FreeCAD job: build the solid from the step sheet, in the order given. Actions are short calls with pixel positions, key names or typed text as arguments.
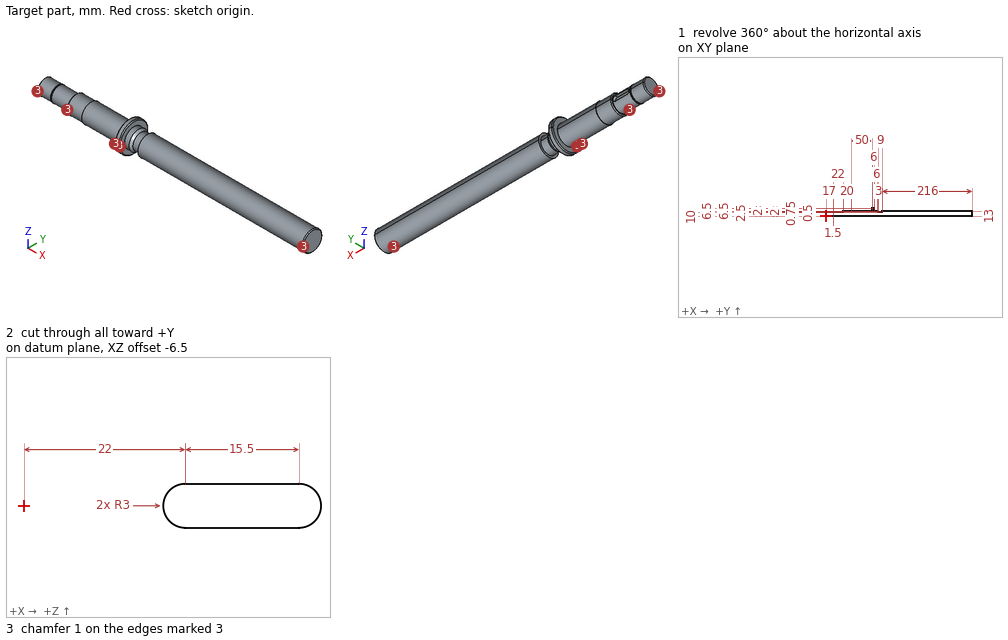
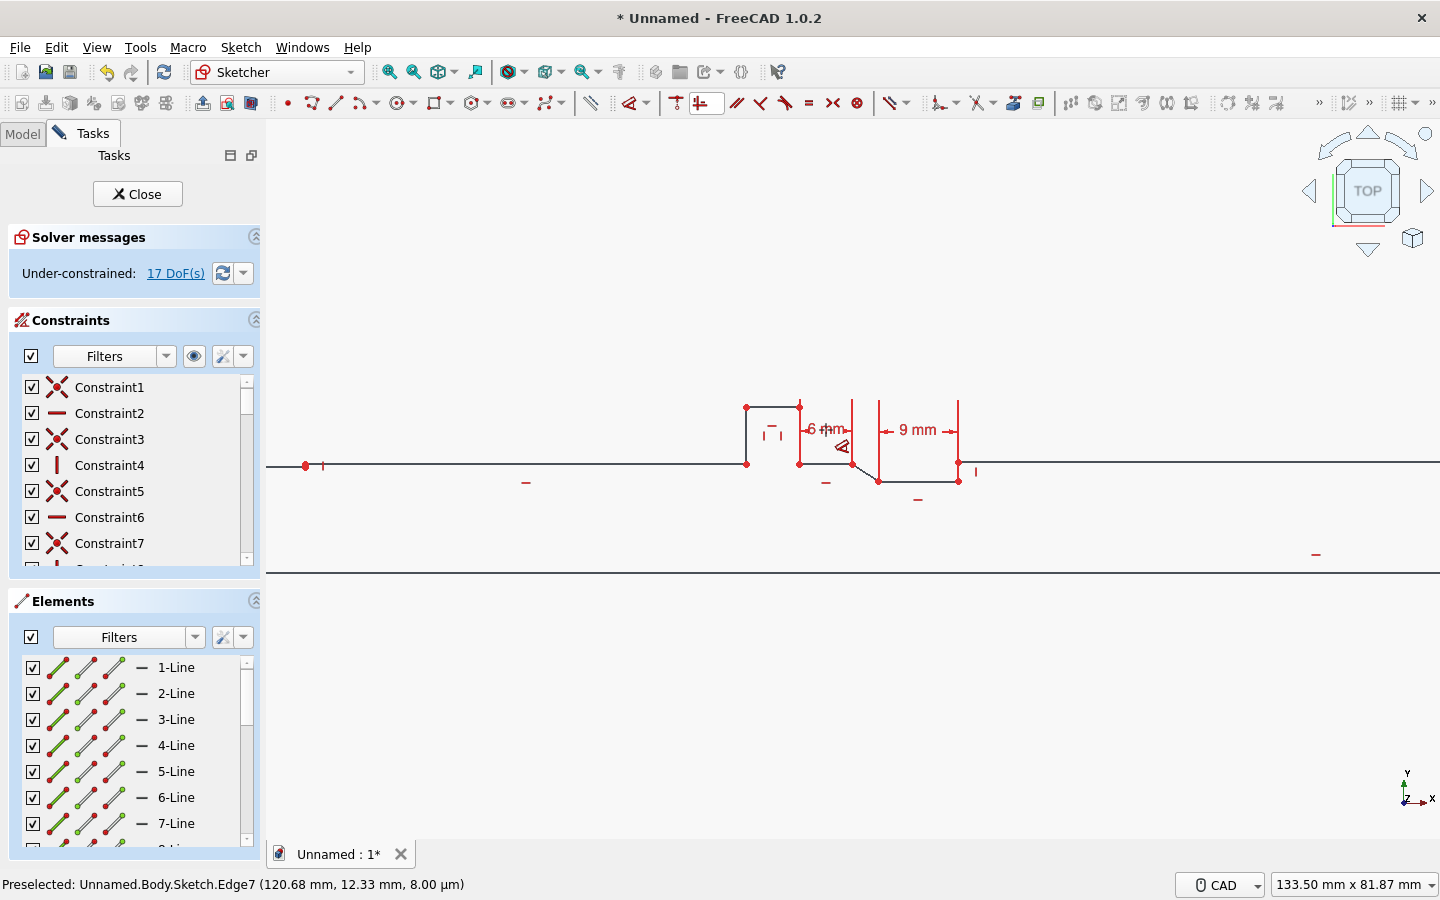
click(784, 407)
click(773, 373)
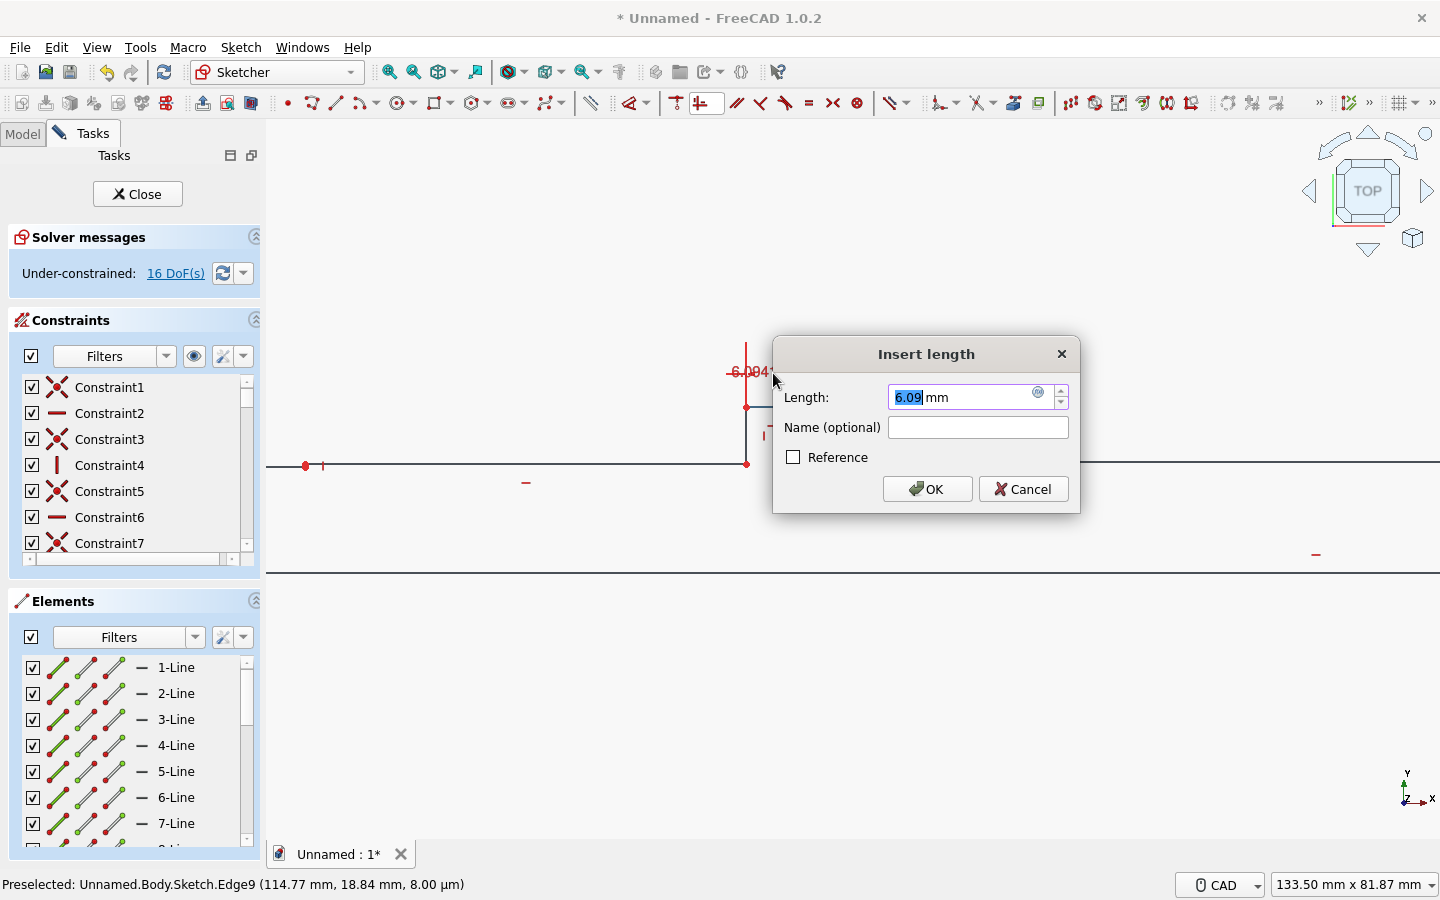
text(6)
key(Return)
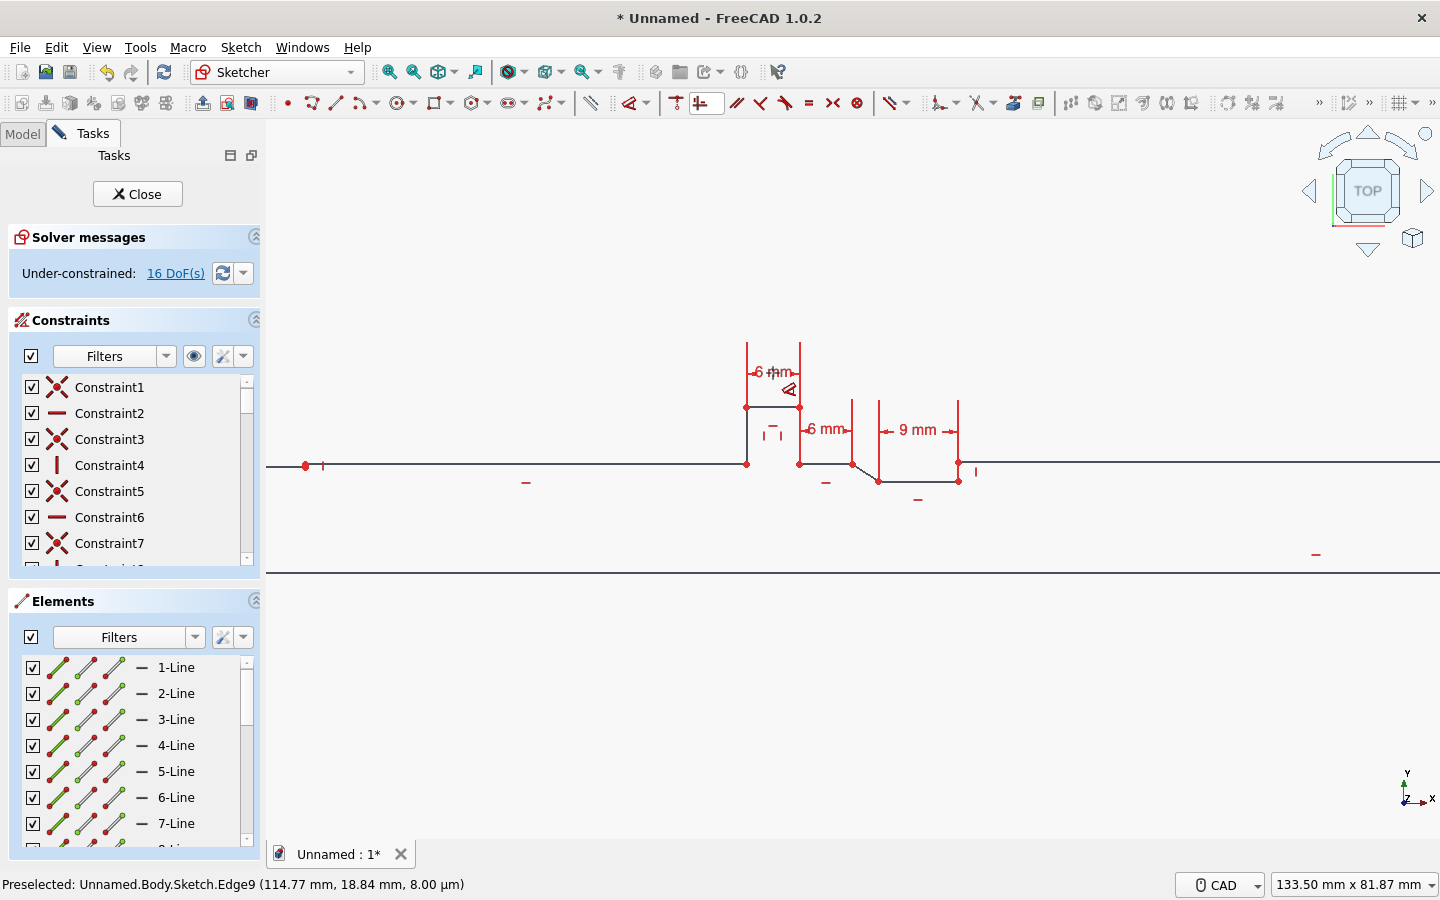
scroll(611, 476, down, 7)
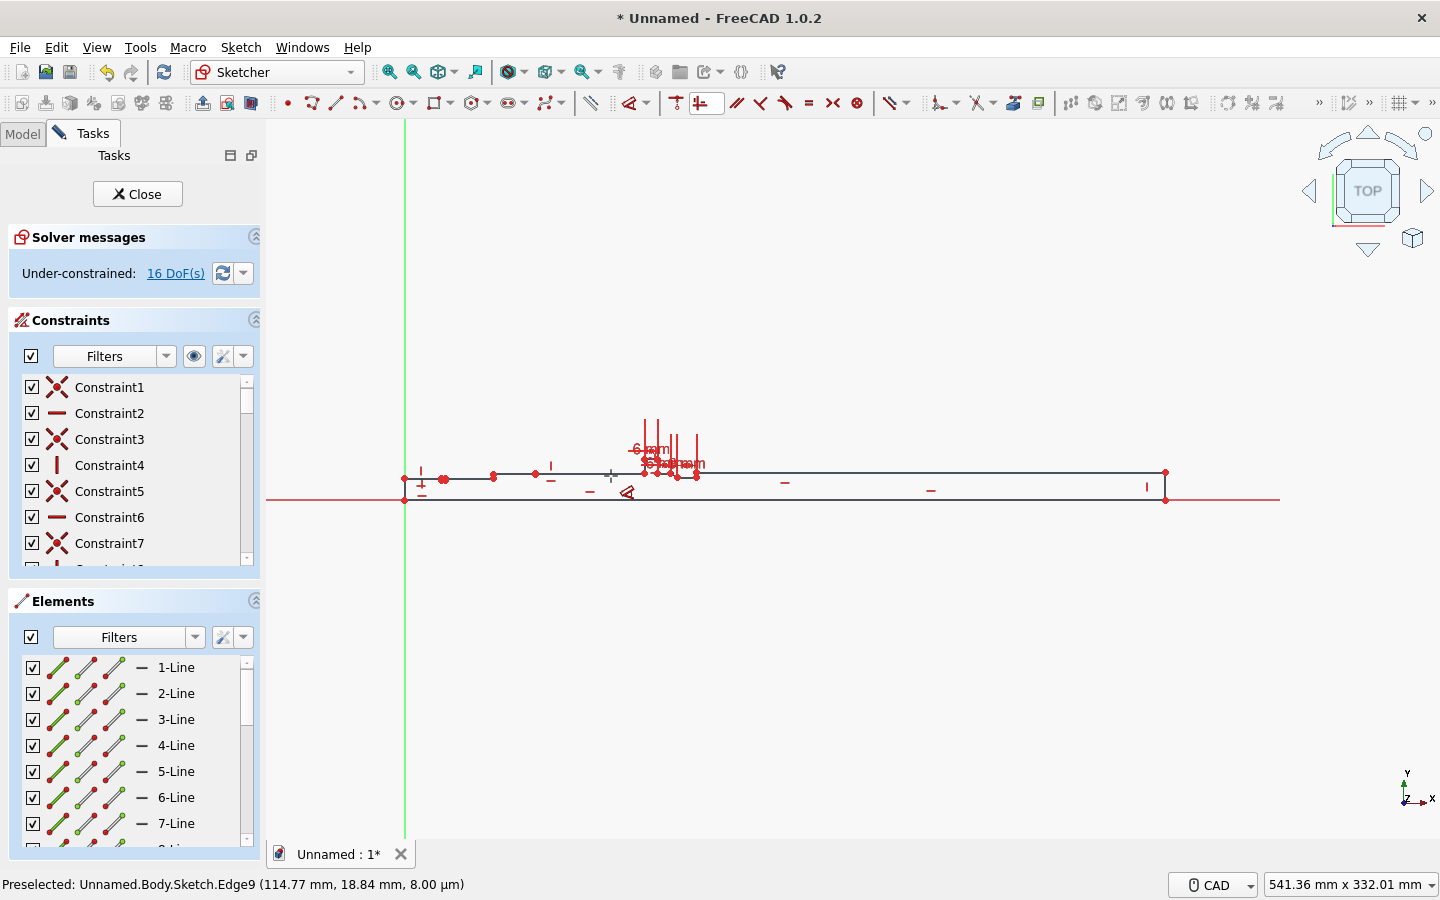
scroll(493, 477, up, 12)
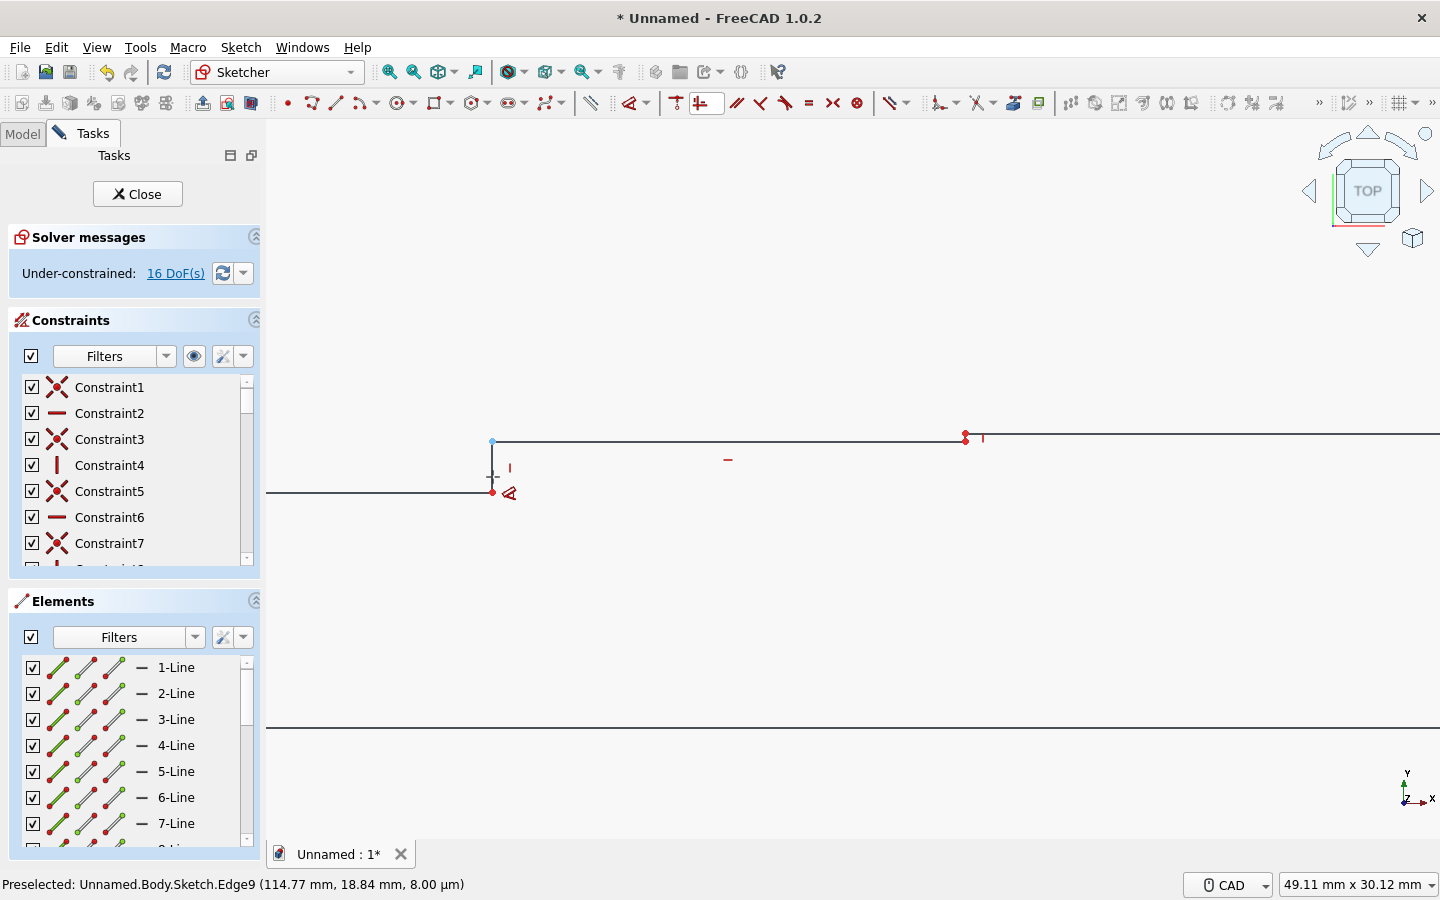
click(492, 467)
click(458, 467)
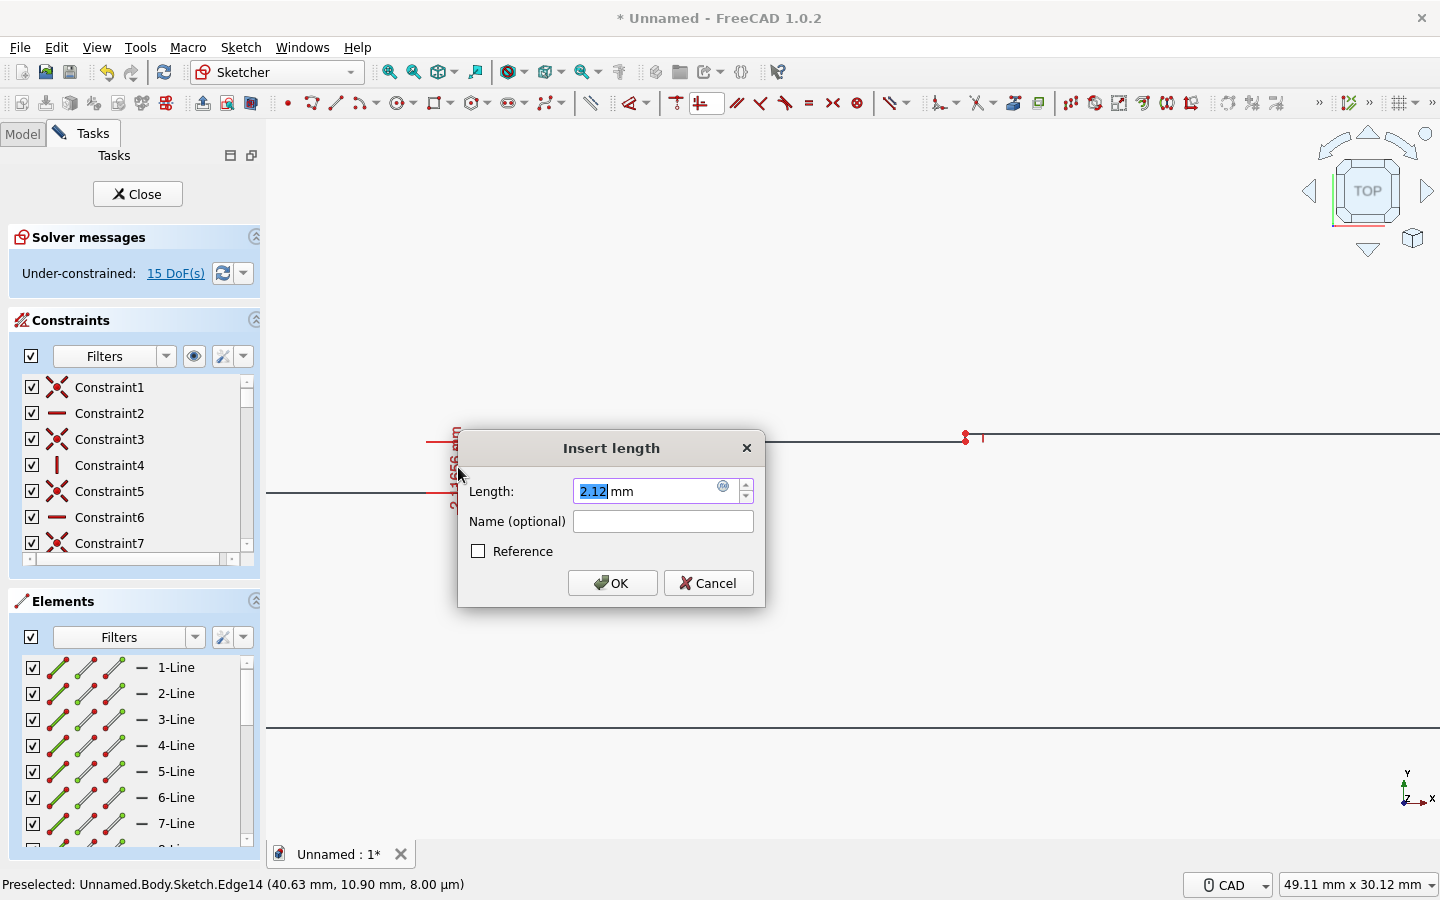
text(2)
key(Return)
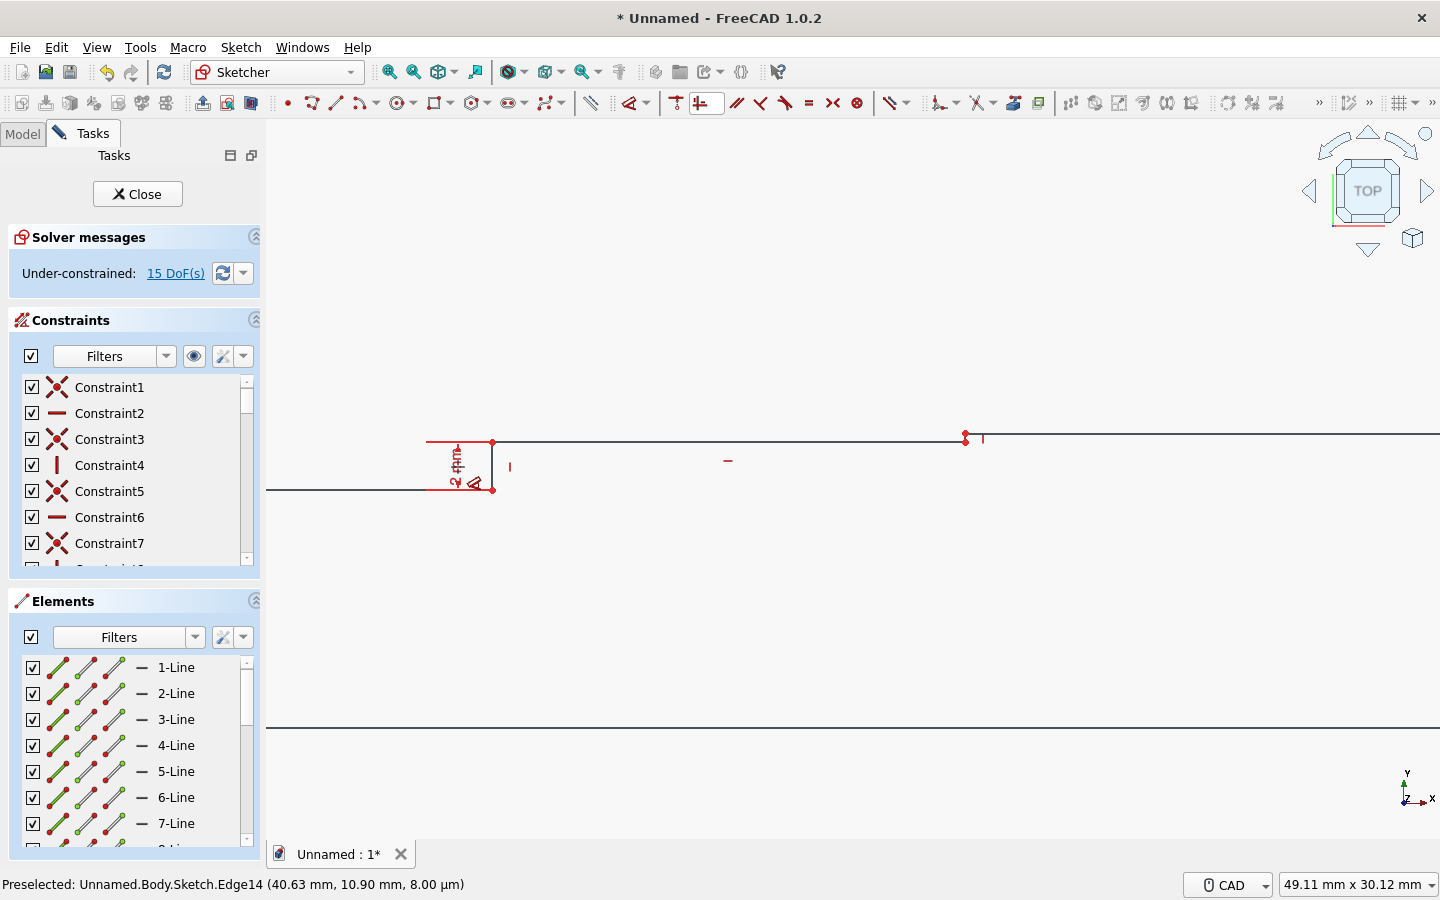
scroll(493, 477, down, 12)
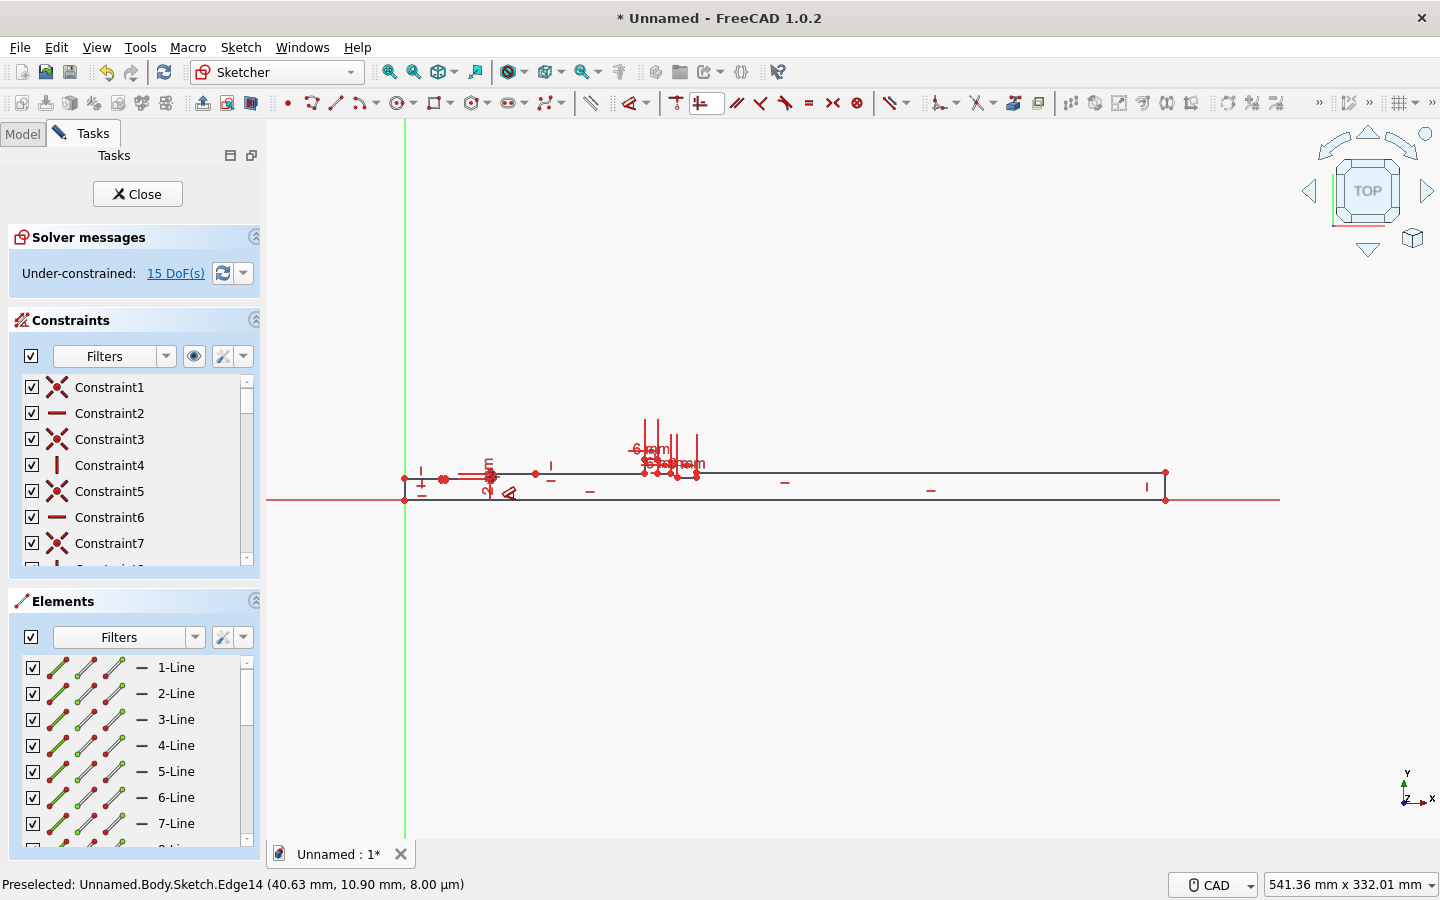
scroll(1165, 492, up, 3)